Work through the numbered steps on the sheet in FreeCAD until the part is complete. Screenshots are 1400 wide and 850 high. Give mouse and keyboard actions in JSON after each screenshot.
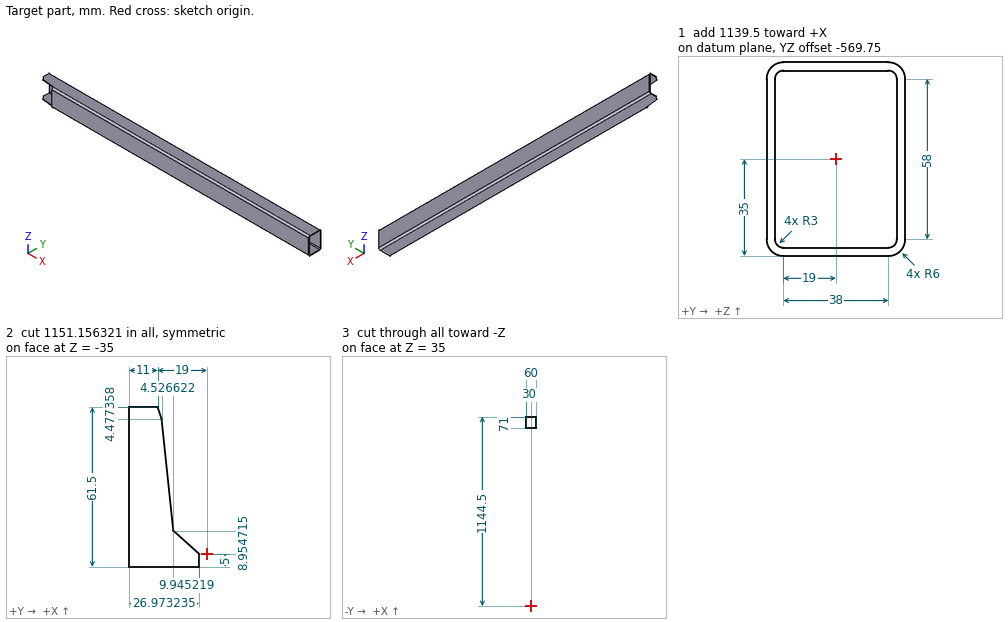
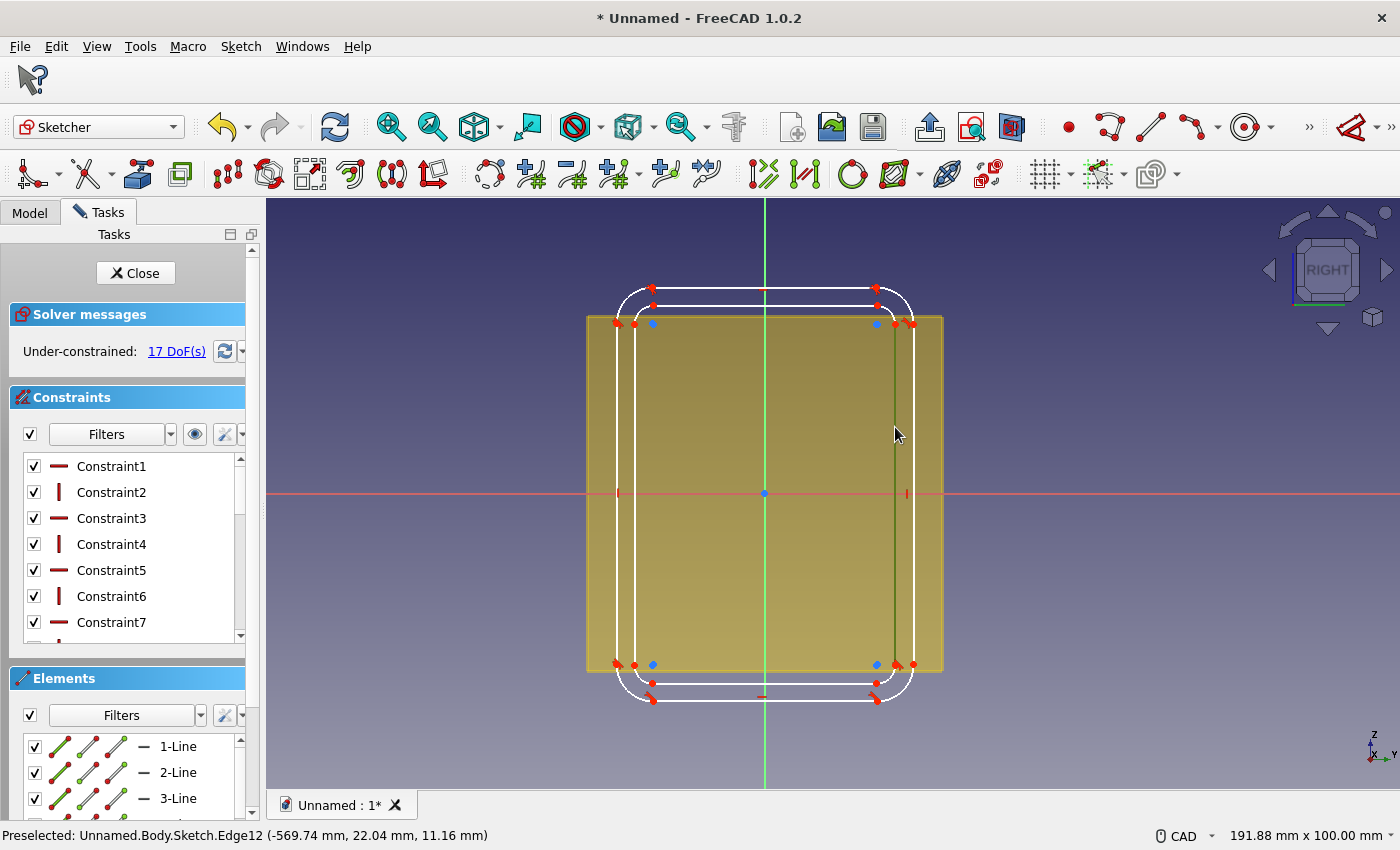
{"action": "left_click", "coordinate": [890, 679]}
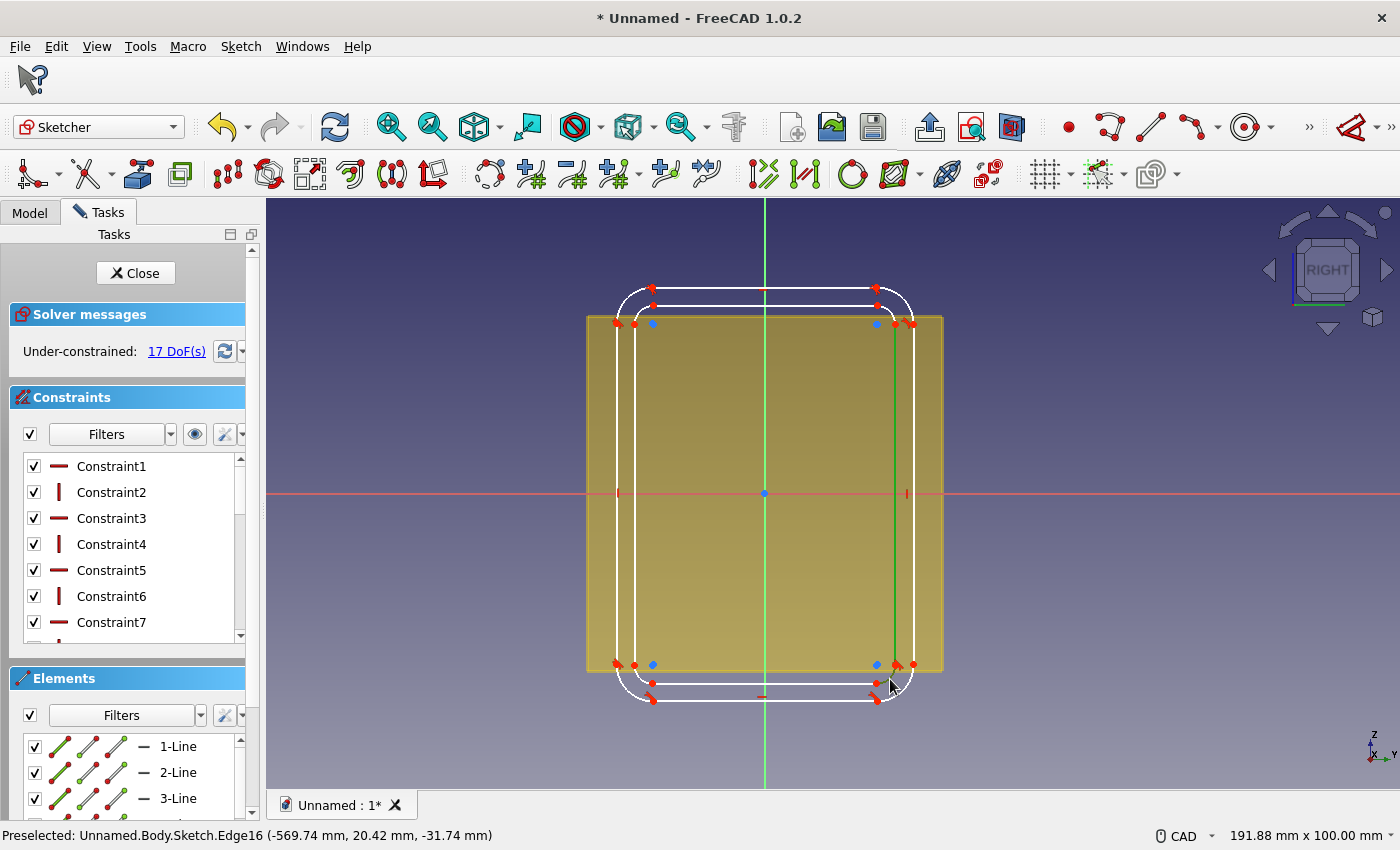
{"action": "key", "text": "t"}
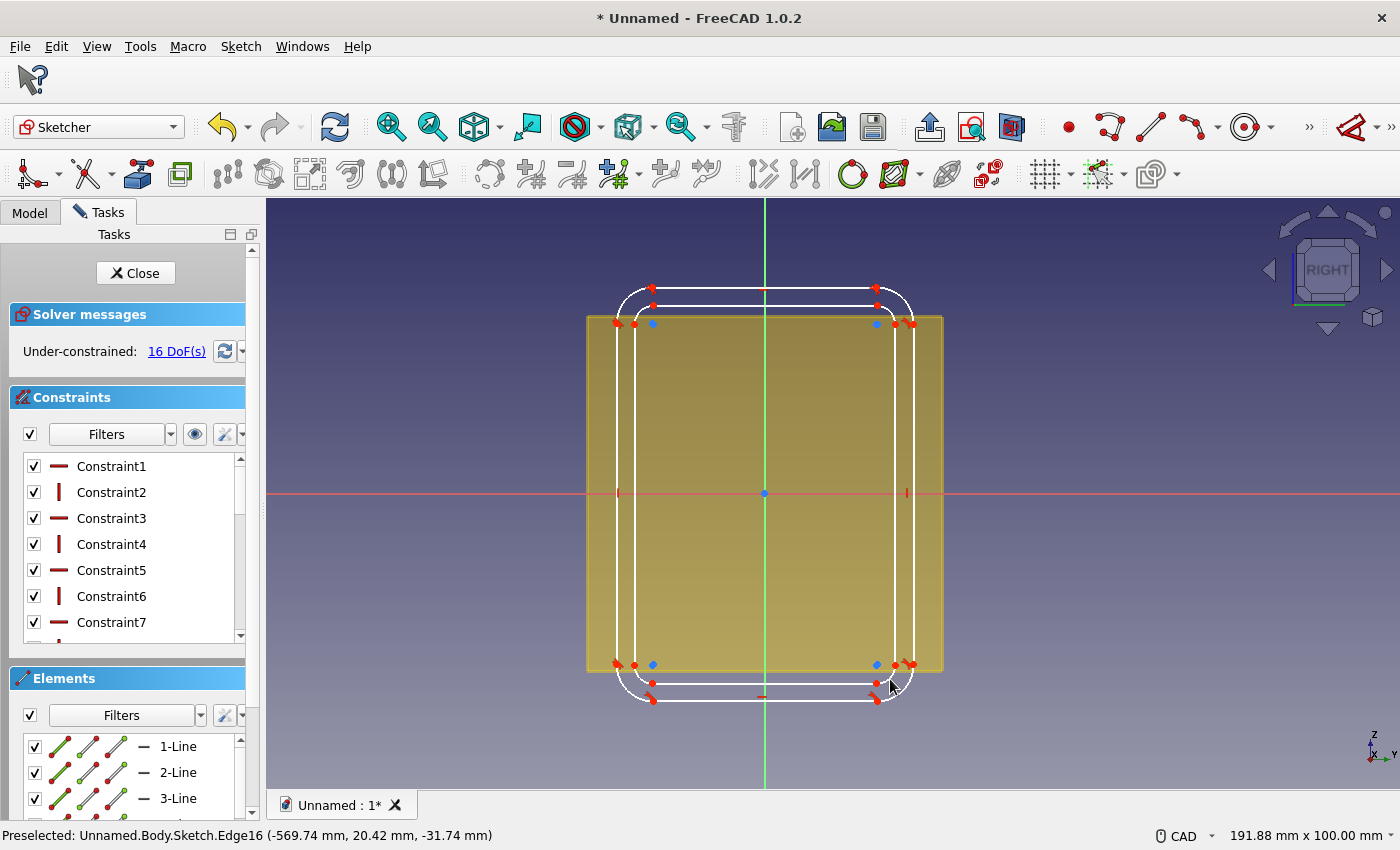
{"action": "left_click", "coordinate": [621, 681]}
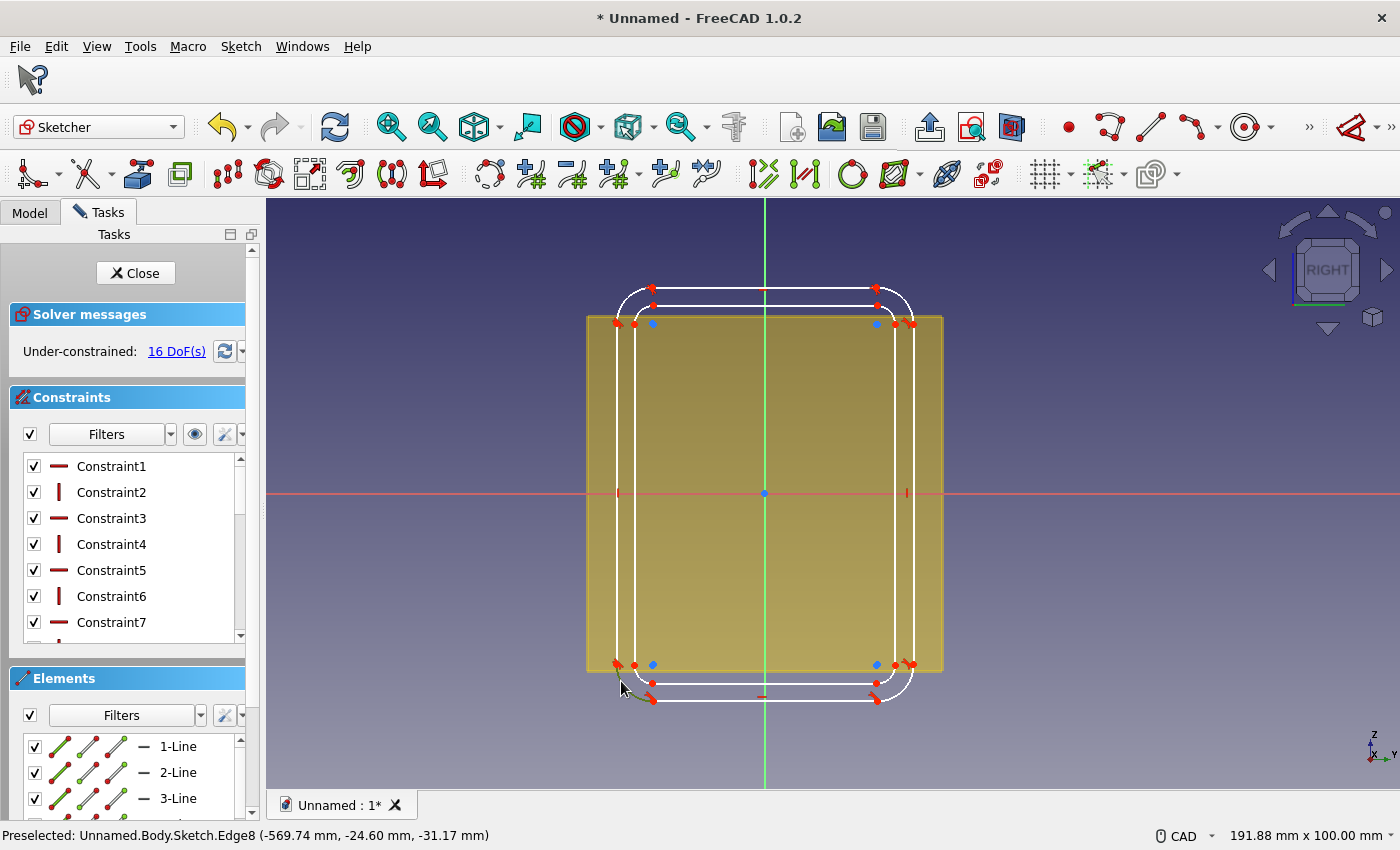
{"action": "left_click", "coordinate": [640, 678]}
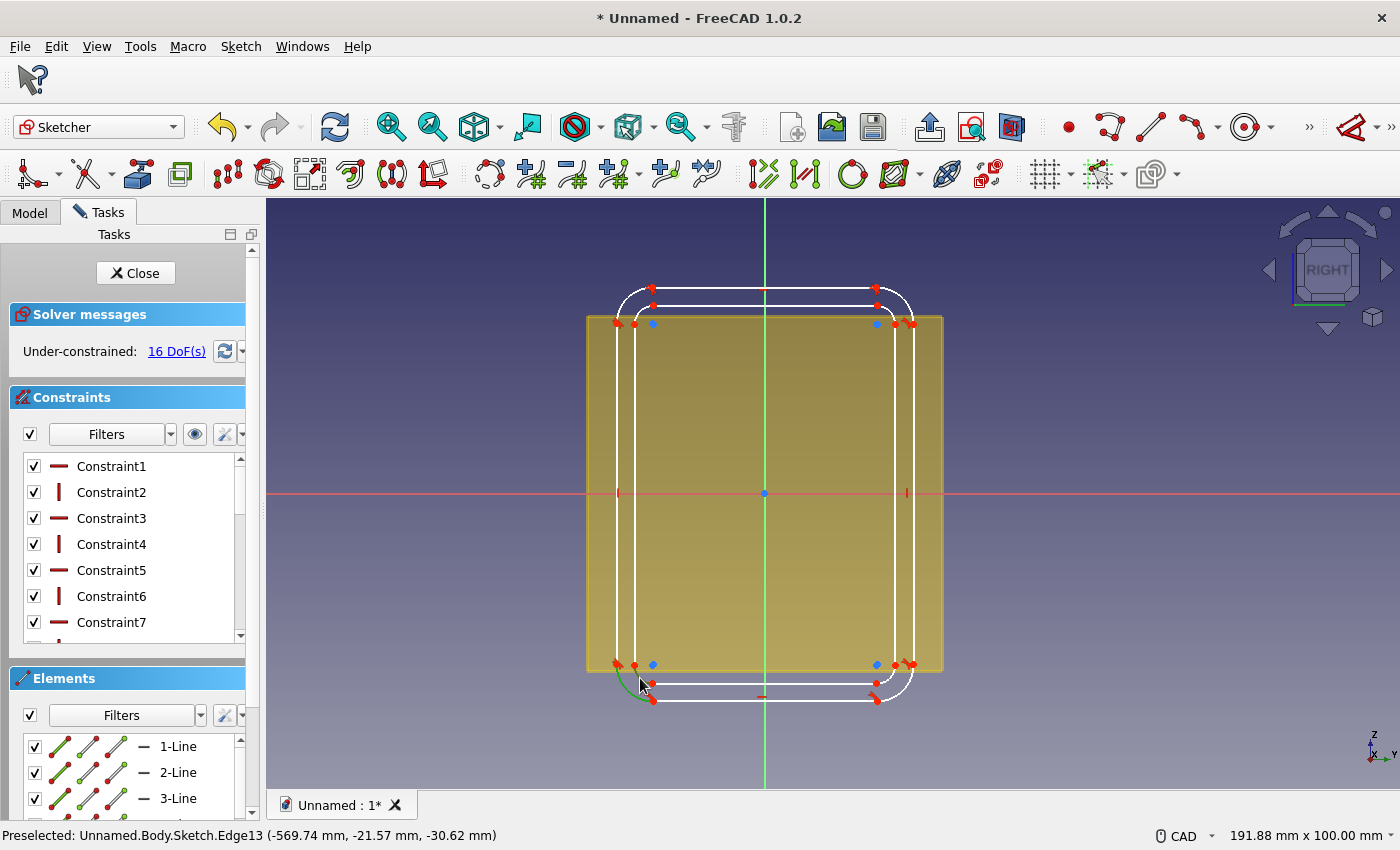
{"action": "key", "text": "c"}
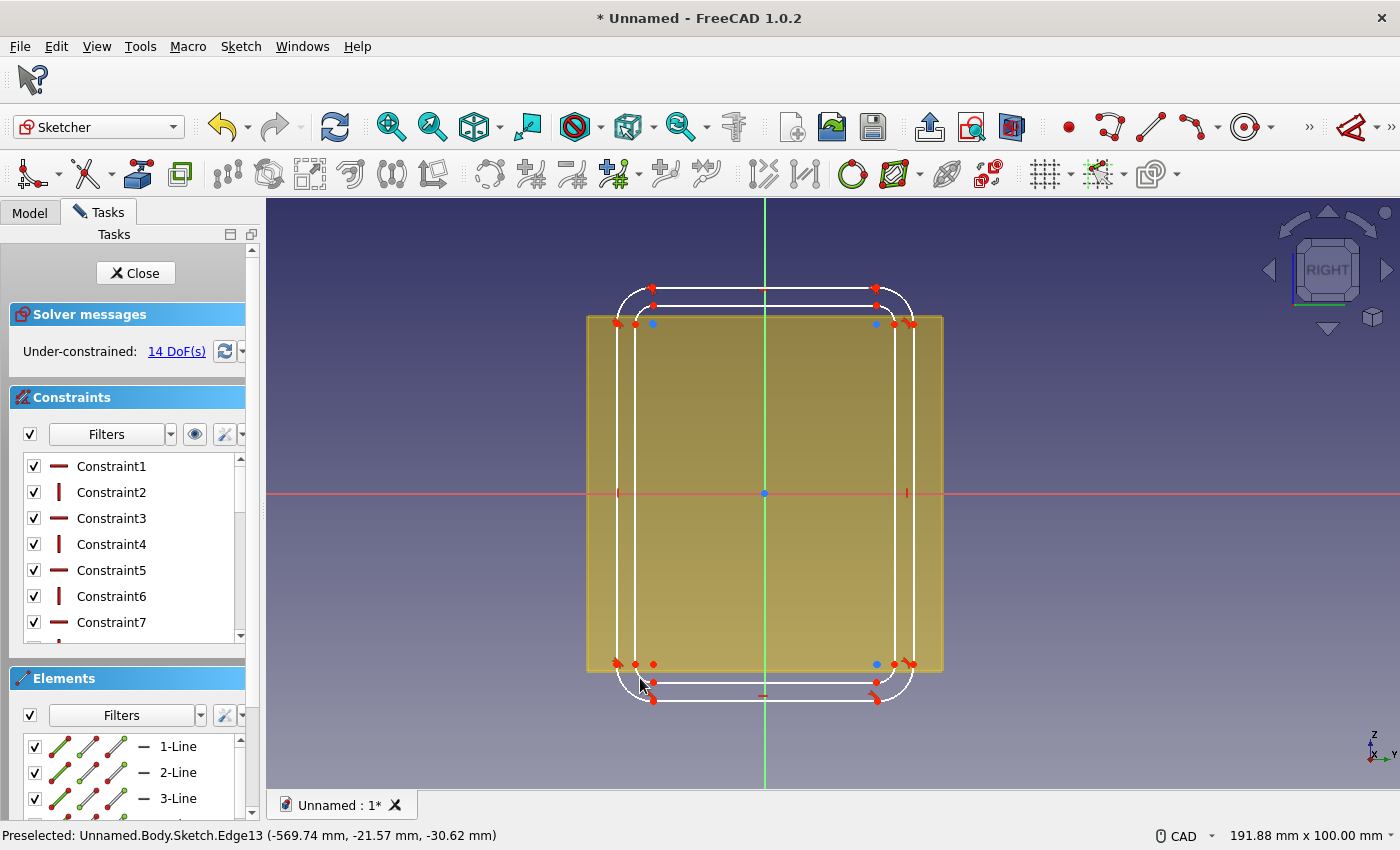
{"action": "left_click", "coordinate": [636, 292]}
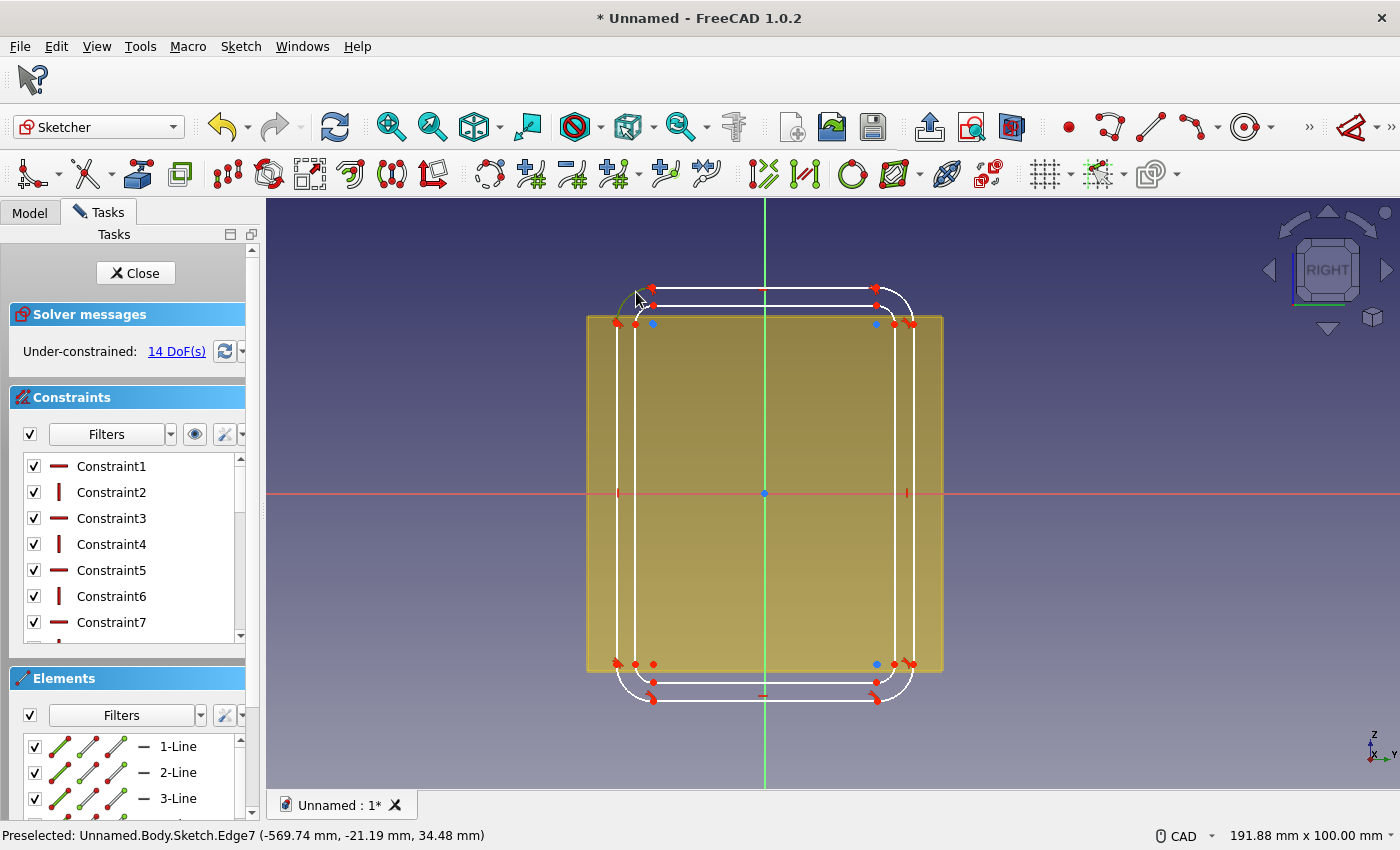
{"action": "left_click", "coordinate": [641, 311]}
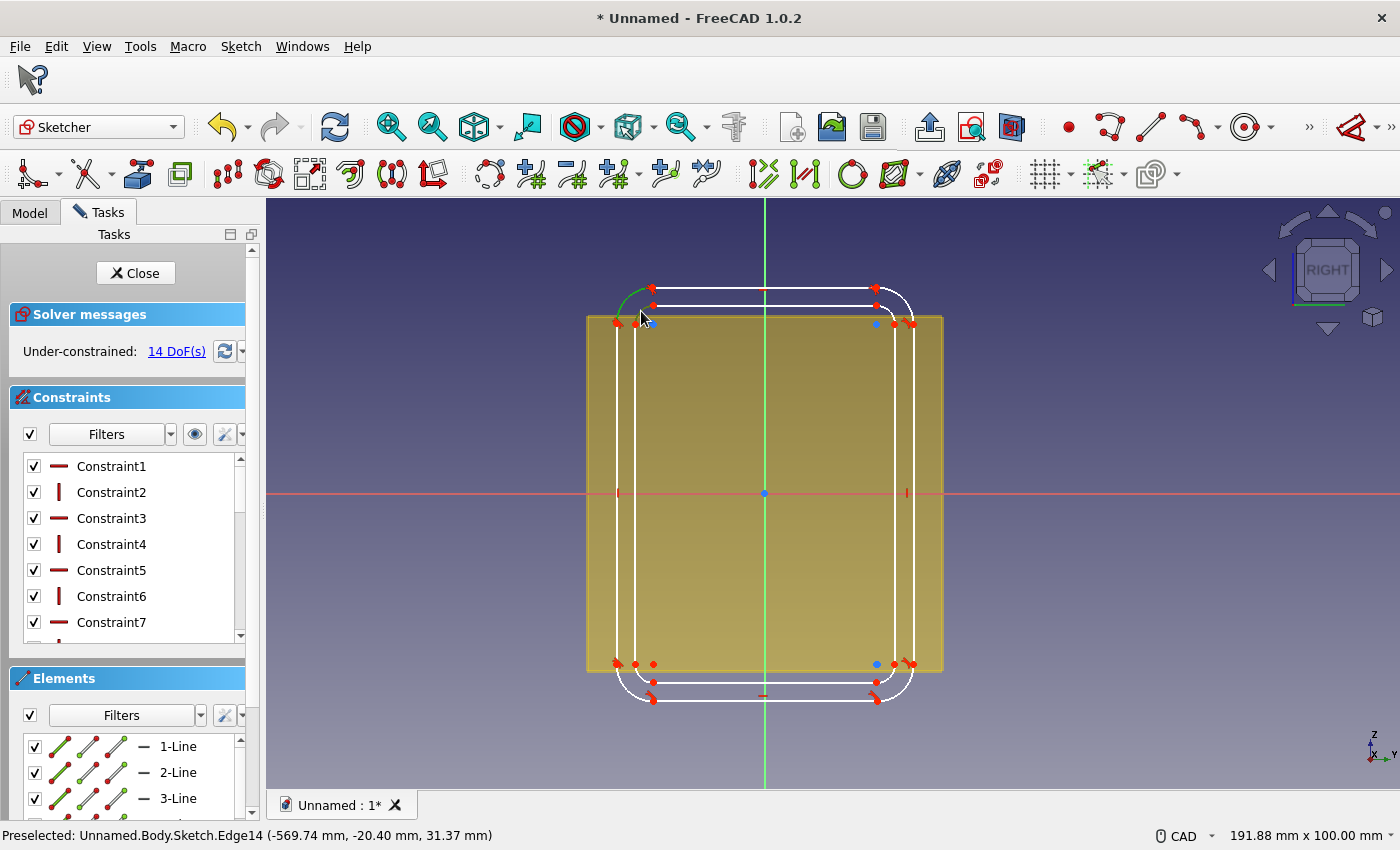
{"action": "key", "text": "c"}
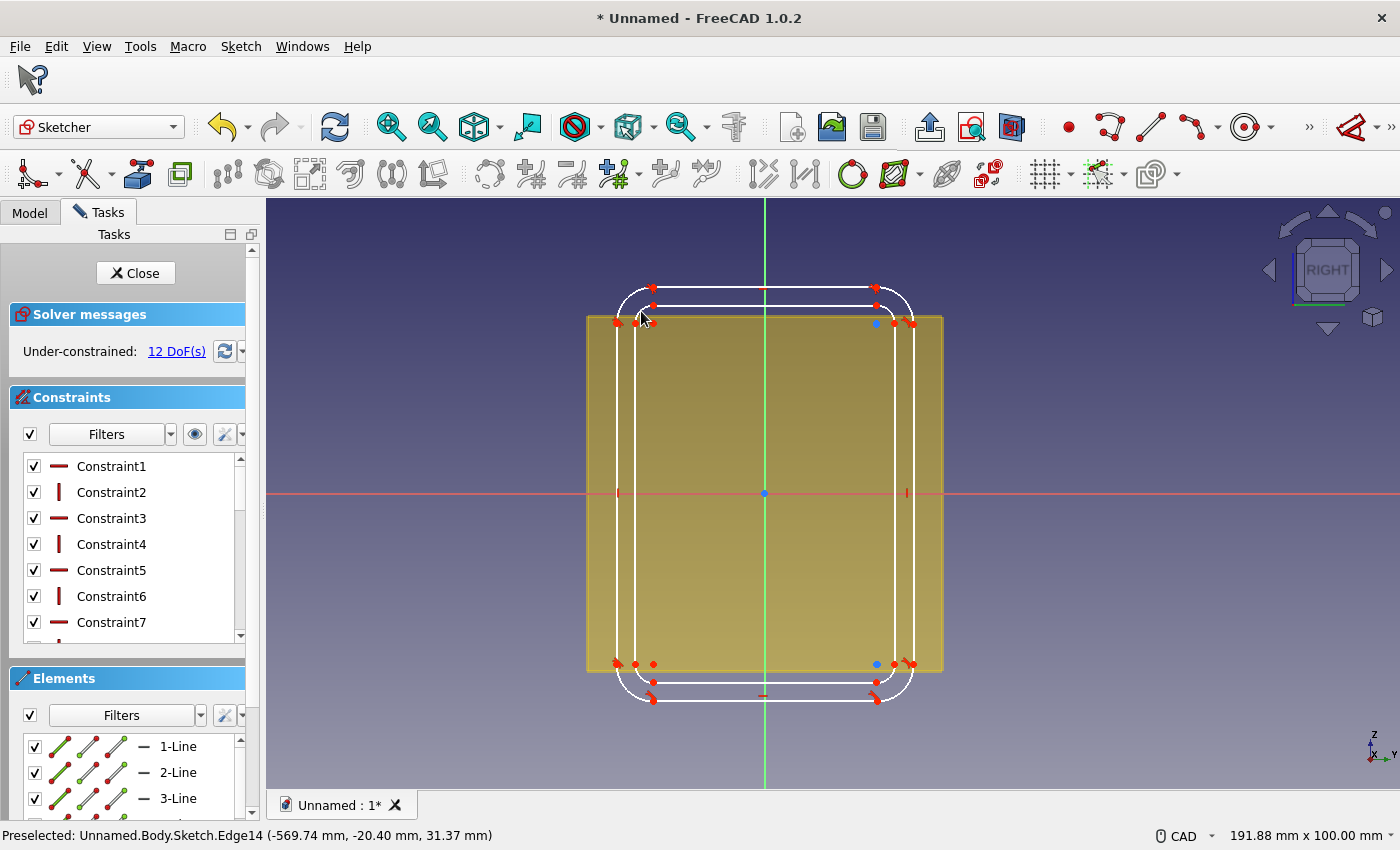
{"action": "left_click", "coordinate": [909, 307]}